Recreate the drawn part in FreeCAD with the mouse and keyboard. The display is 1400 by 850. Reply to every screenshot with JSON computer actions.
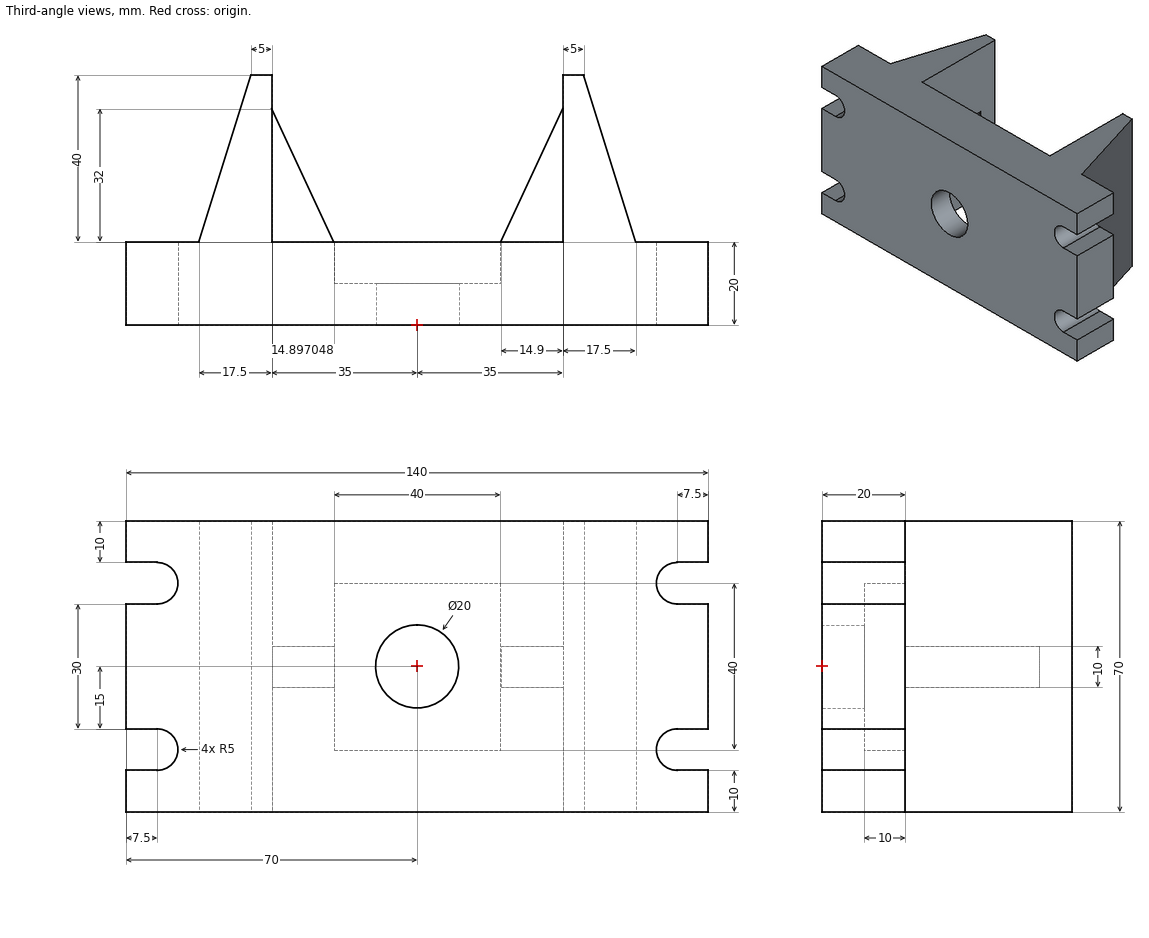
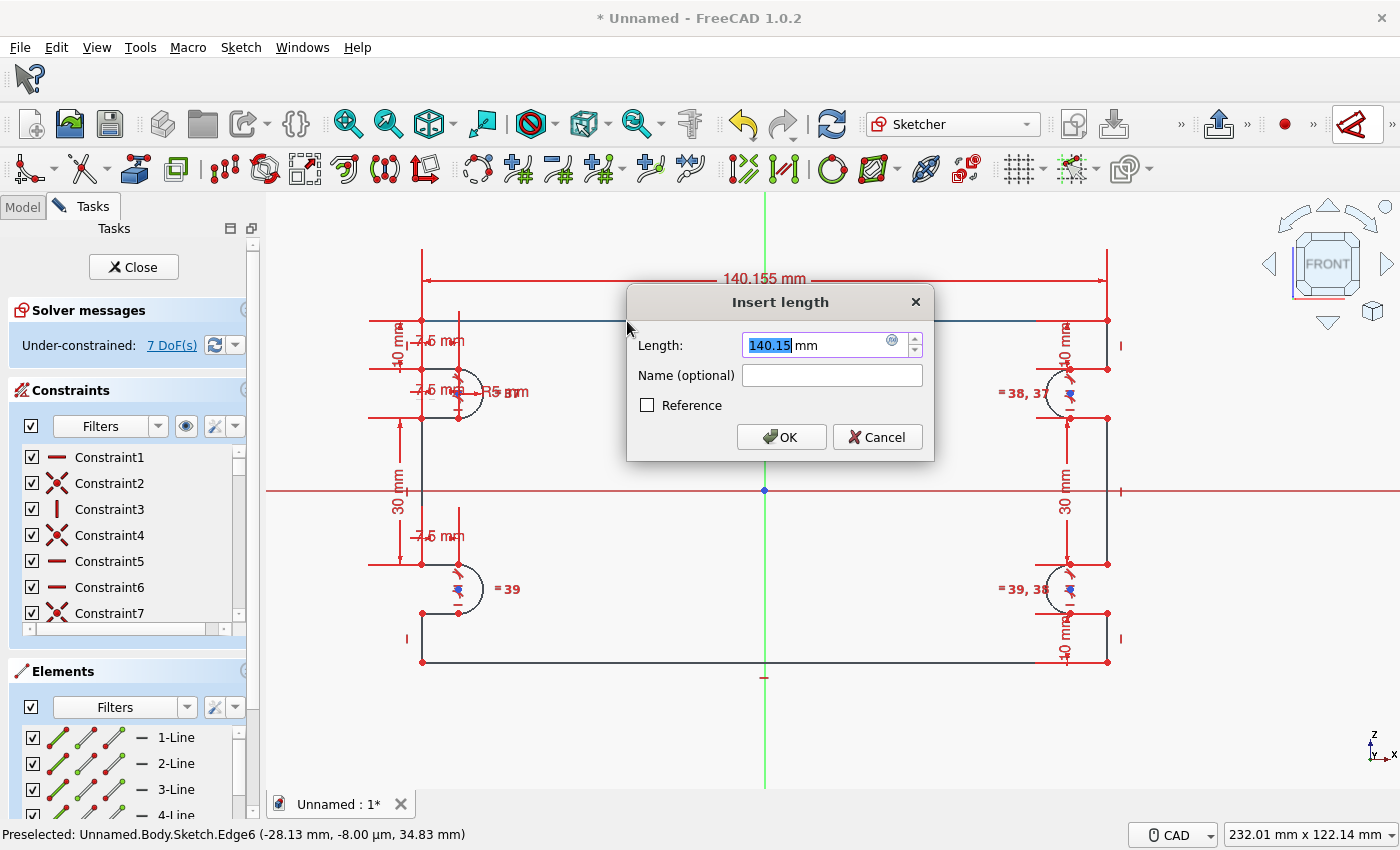
{"action": "type", "text": "140"}
{"action": "key", "text": "Return"}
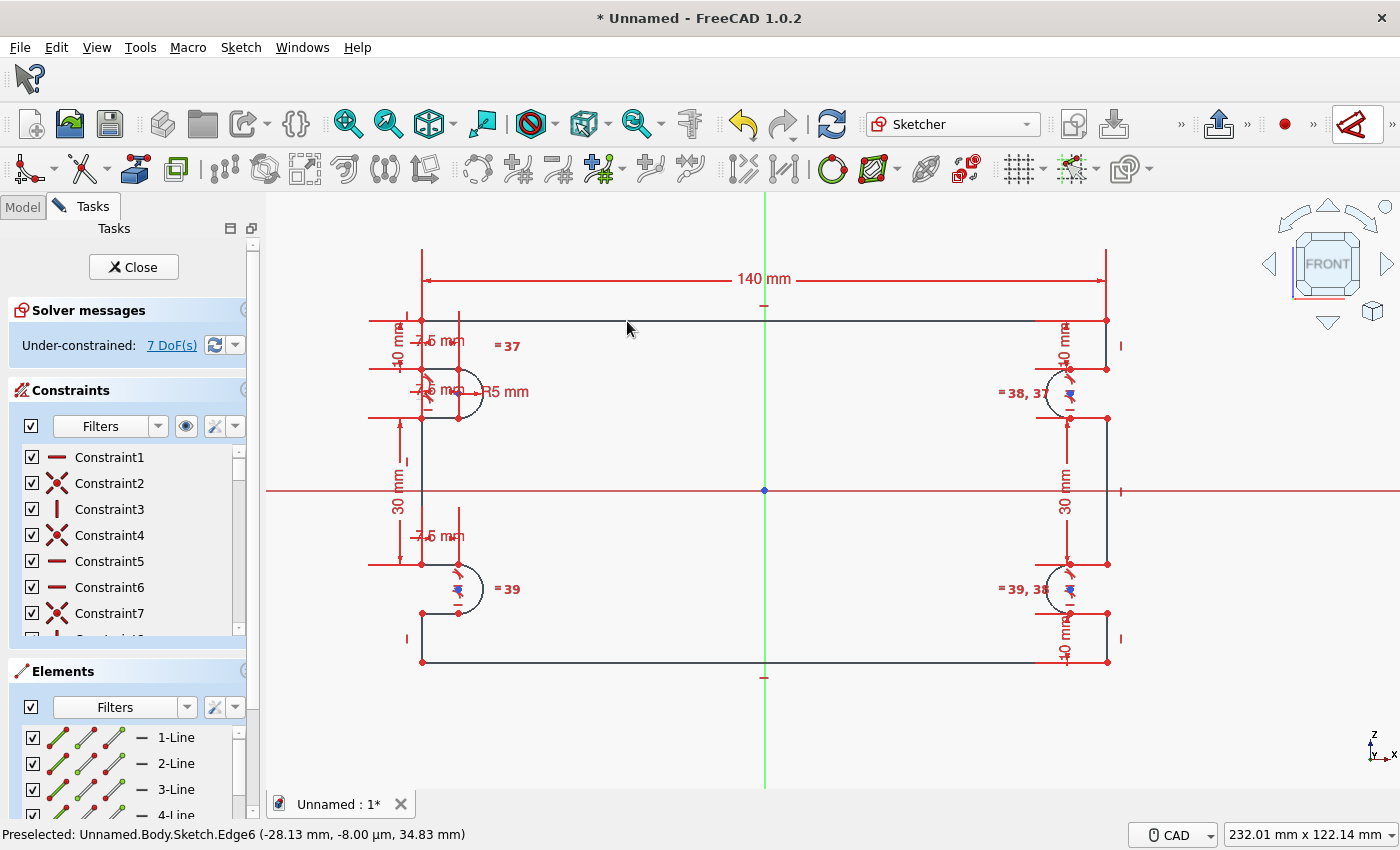
{"action": "scroll", "coordinate": [1096, 369], "scroll_direction": "up", "scroll_amount": 2}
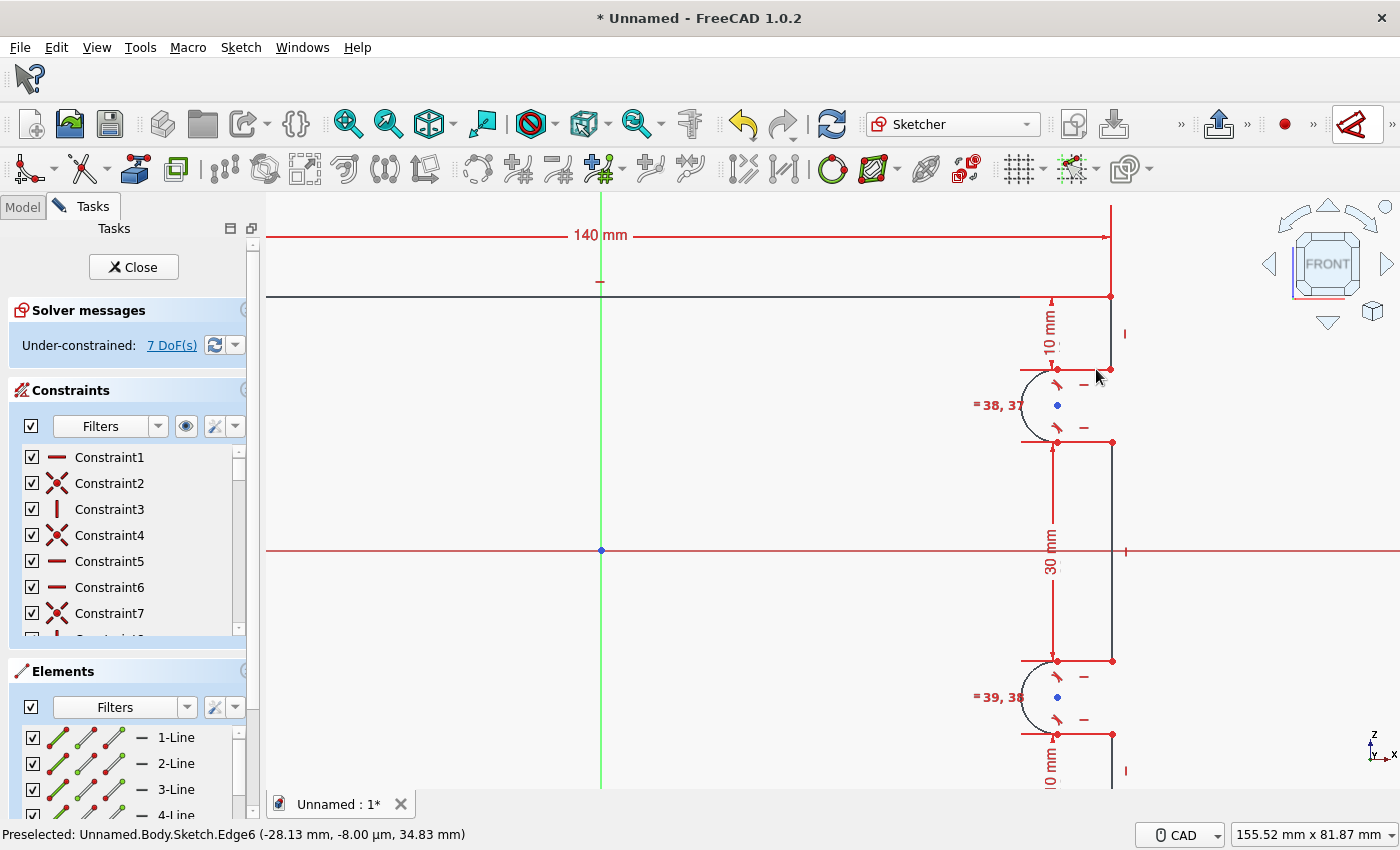
{"action": "left_click", "coordinate": [1095, 370]}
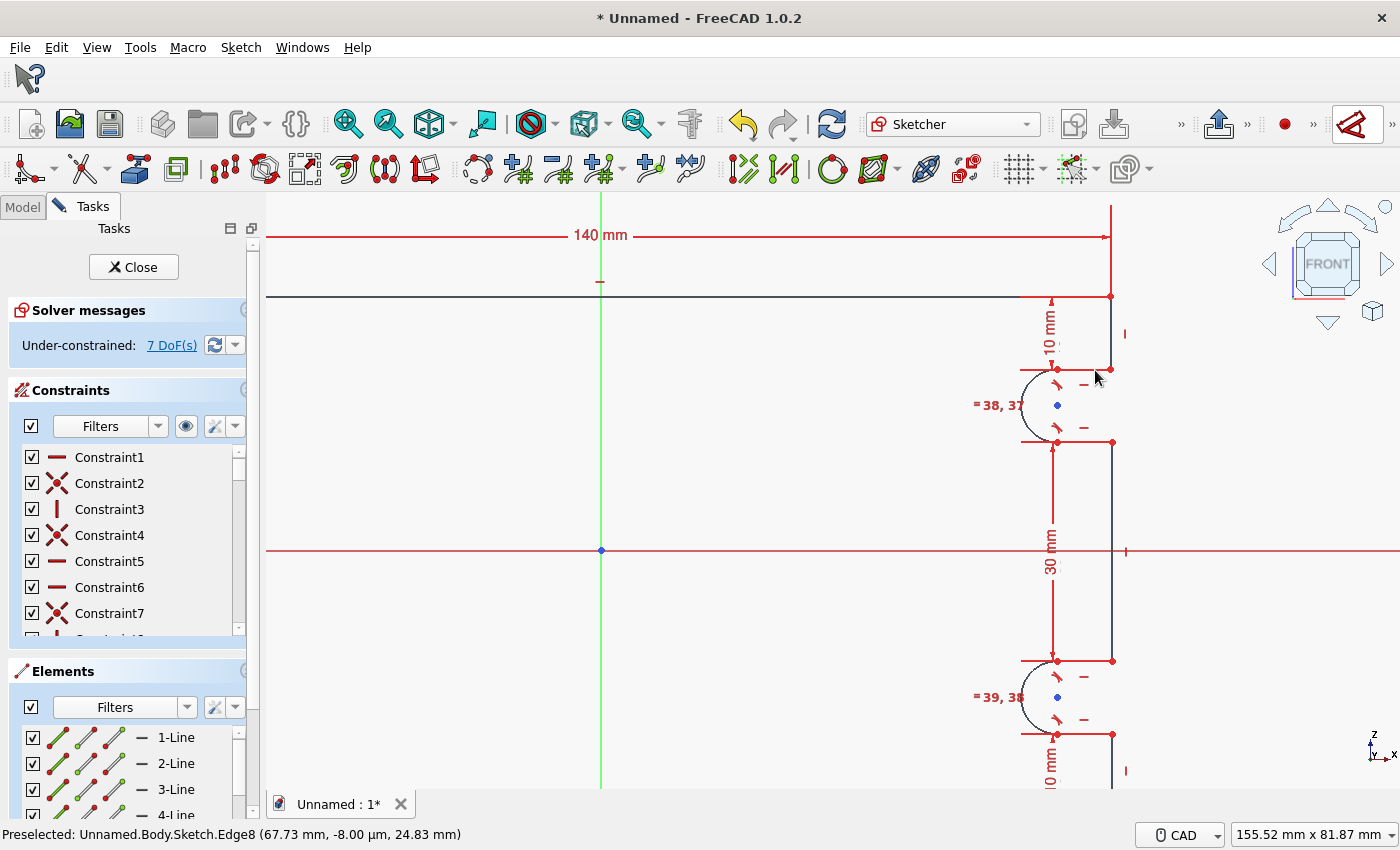
{"action": "left_click", "coordinate": [1378, 124]}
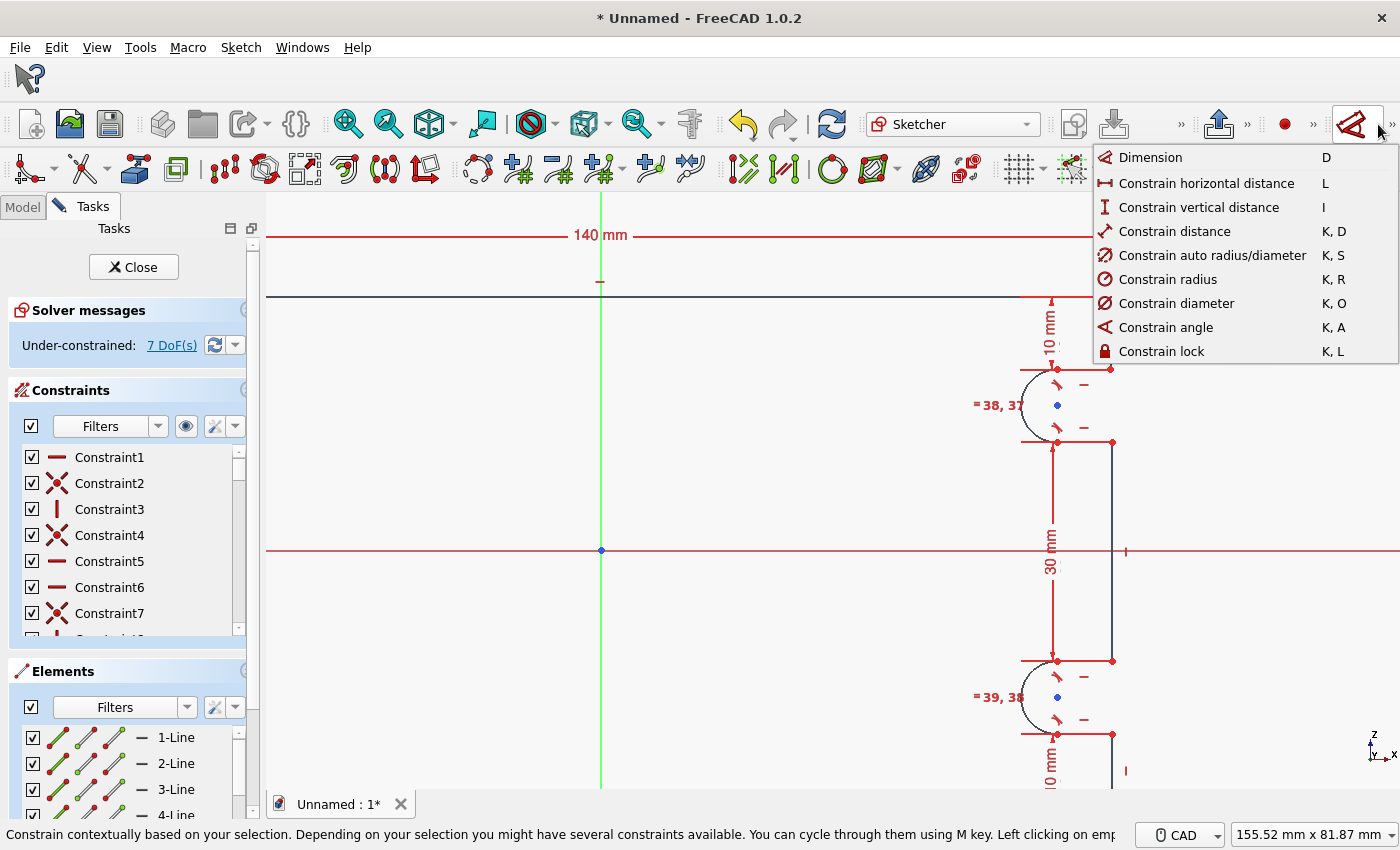
{"action": "left_click", "coordinate": [1246, 183]}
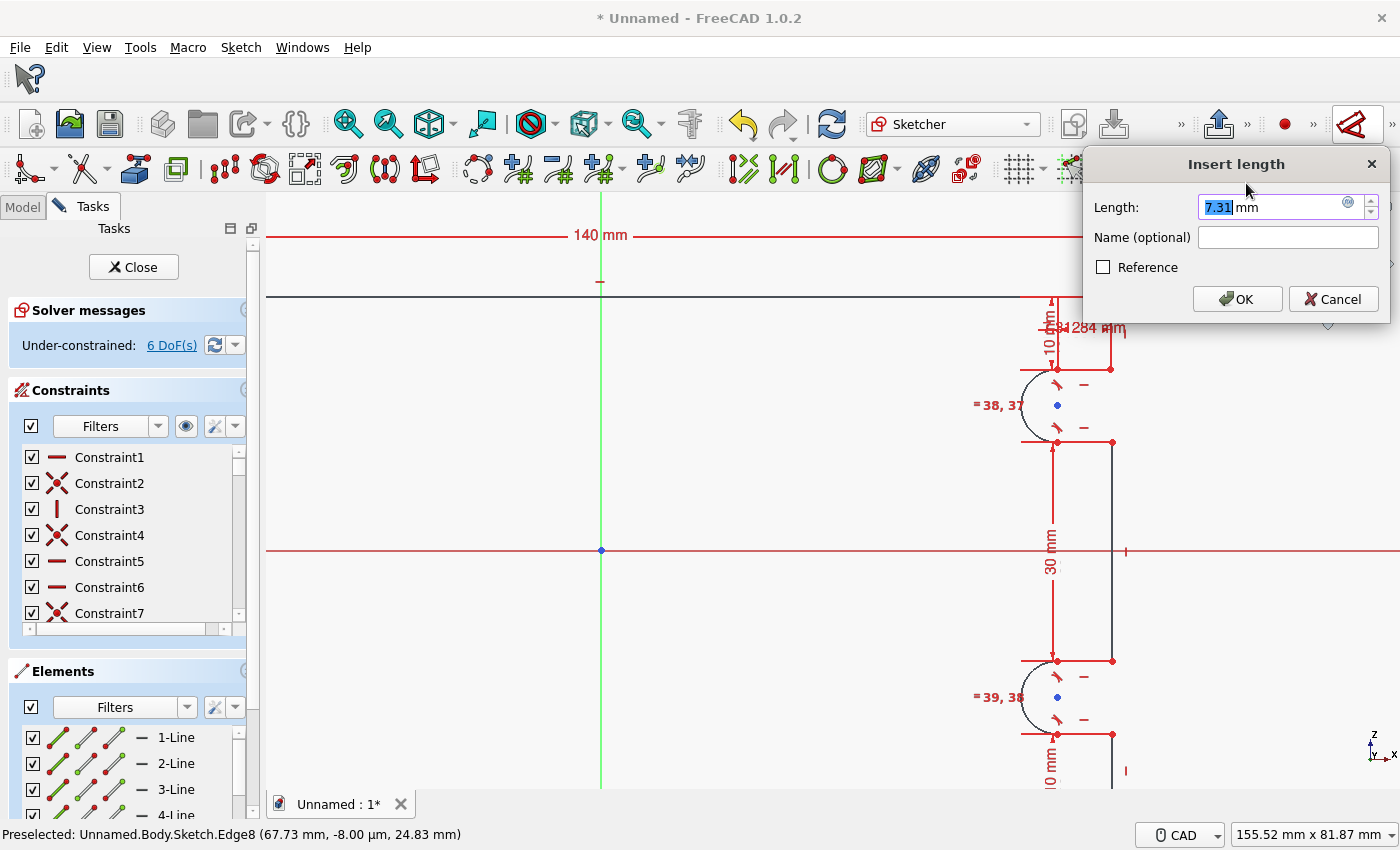
{"action": "type", "text": "7.5"}
{"action": "key", "text": "Return"}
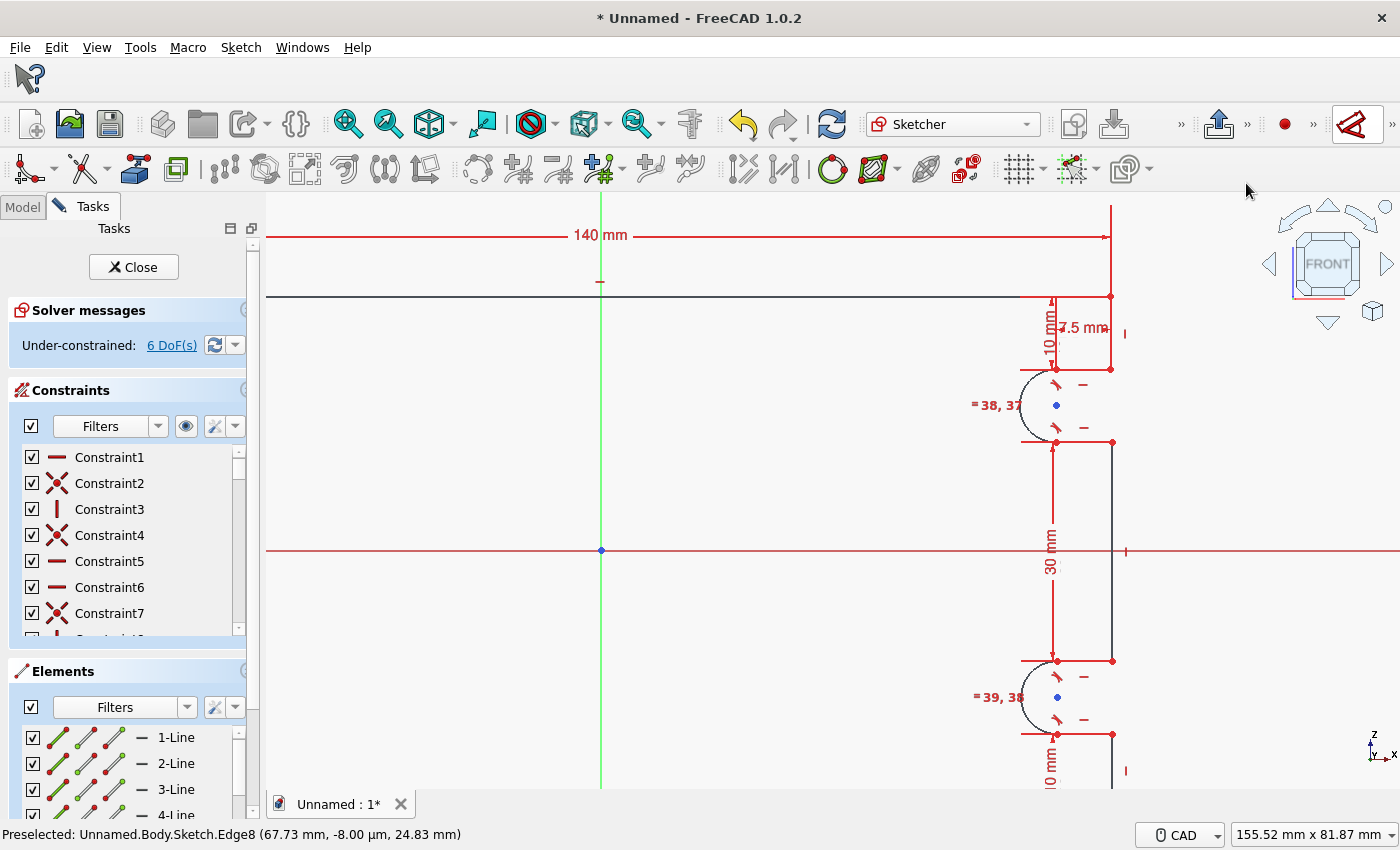
{"action": "left_click", "coordinate": [1073, 442]}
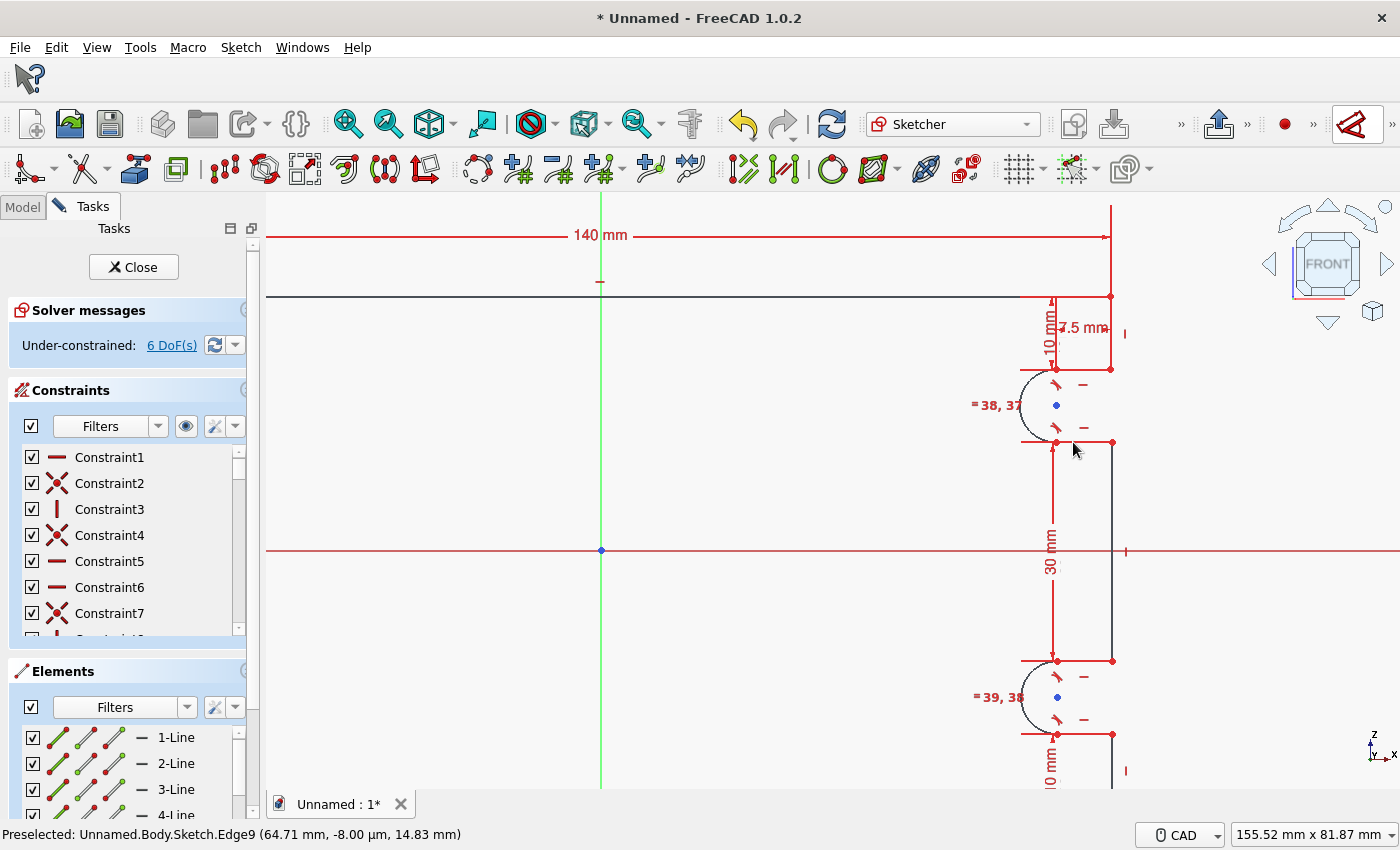
{"action": "key", "text": "l"}